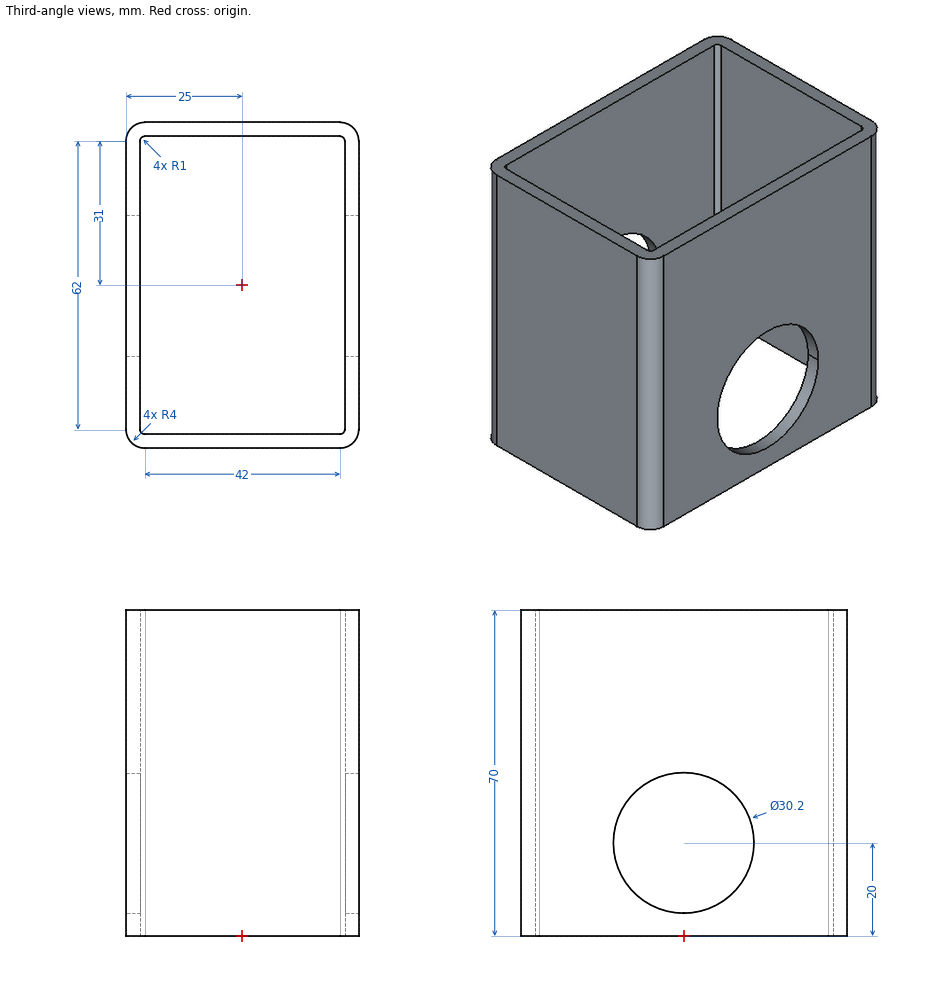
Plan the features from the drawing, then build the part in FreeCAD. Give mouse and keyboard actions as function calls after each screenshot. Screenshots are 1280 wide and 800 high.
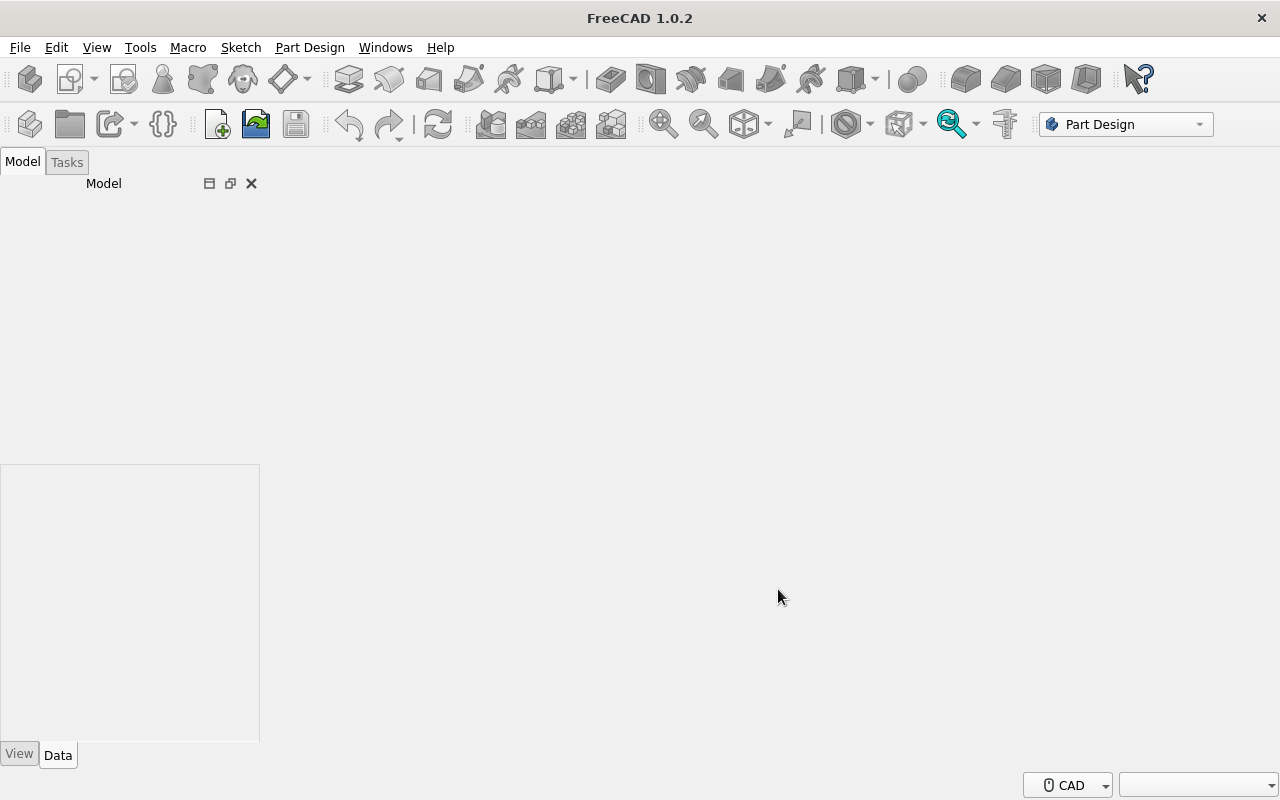
click(216, 124)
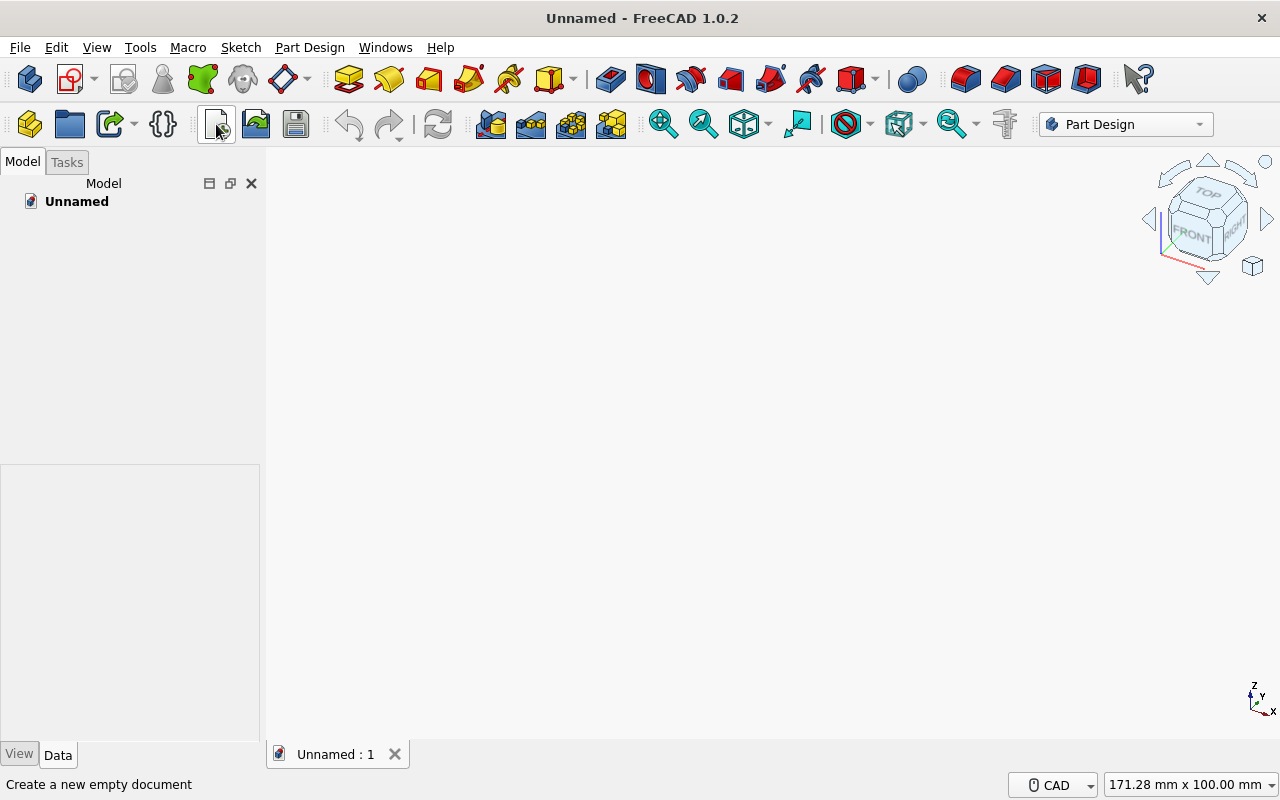
click(70, 80)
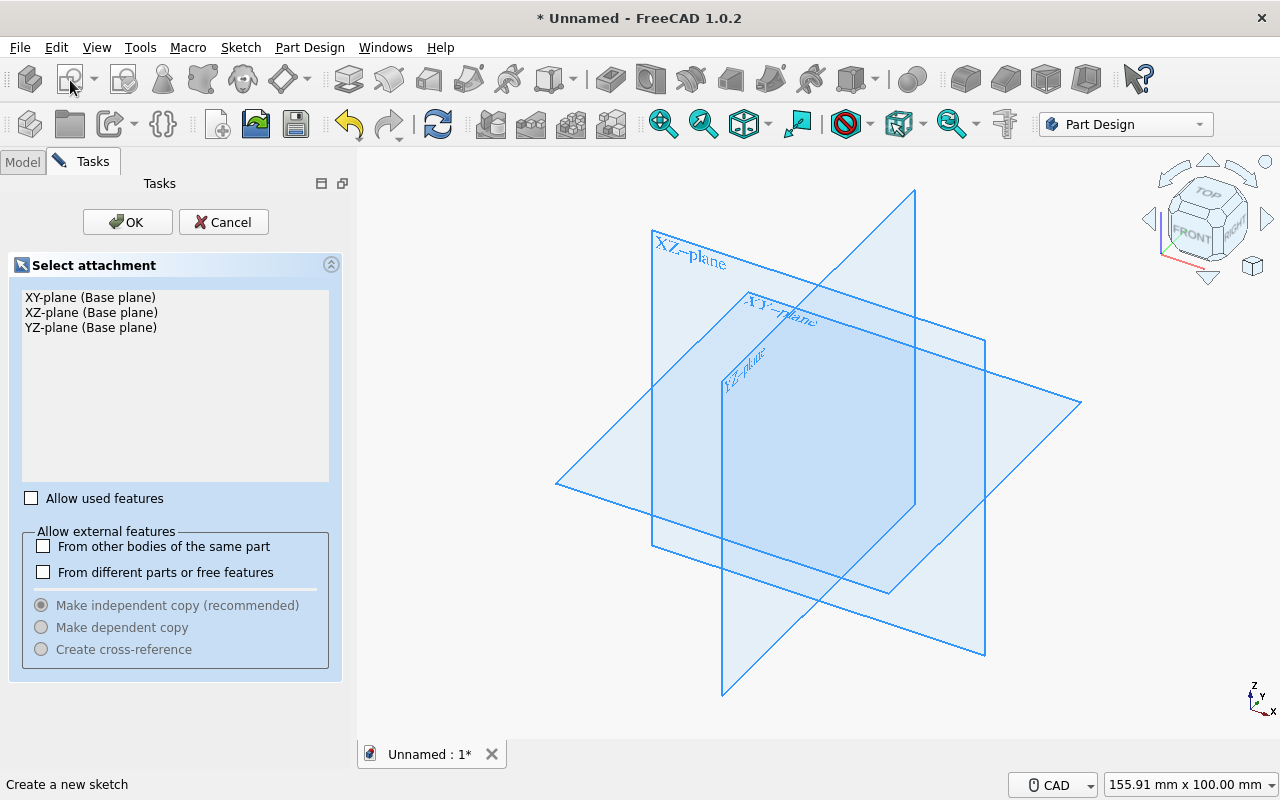
click(82, 298)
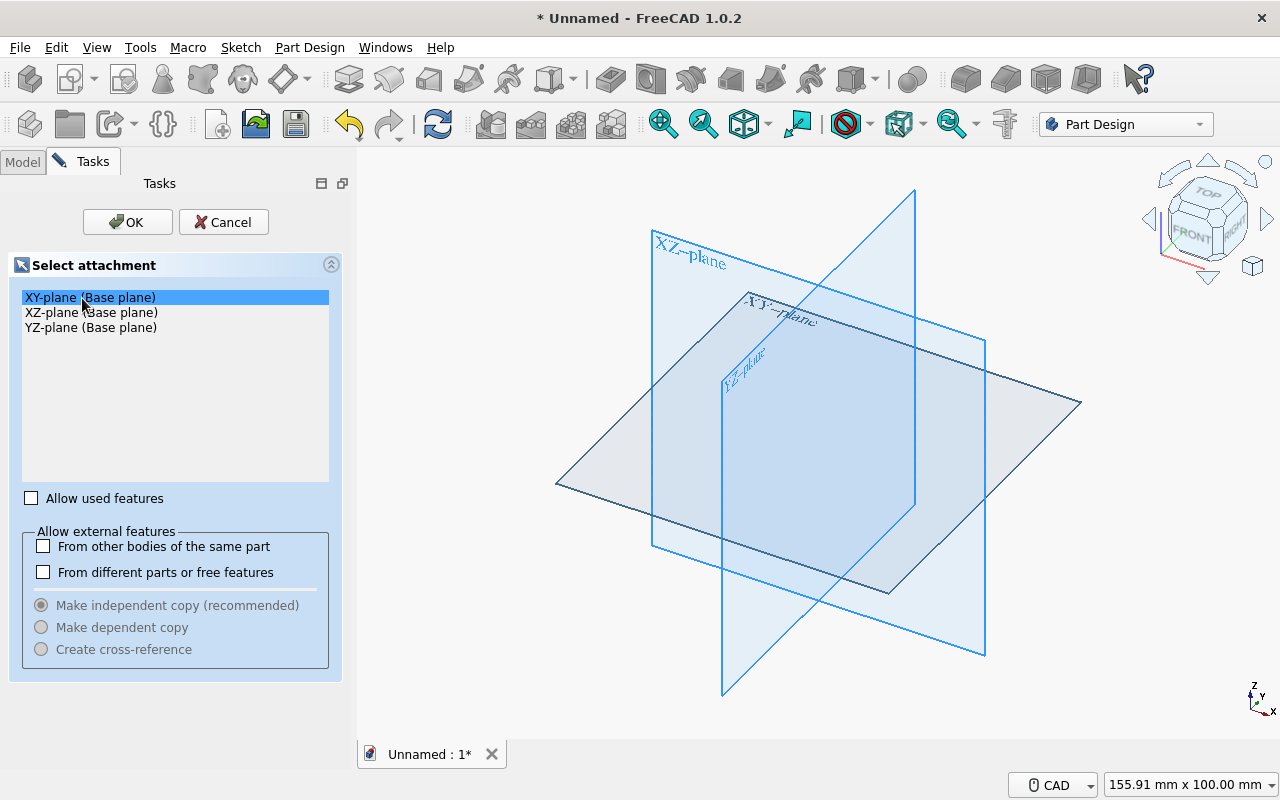
click(128, 222)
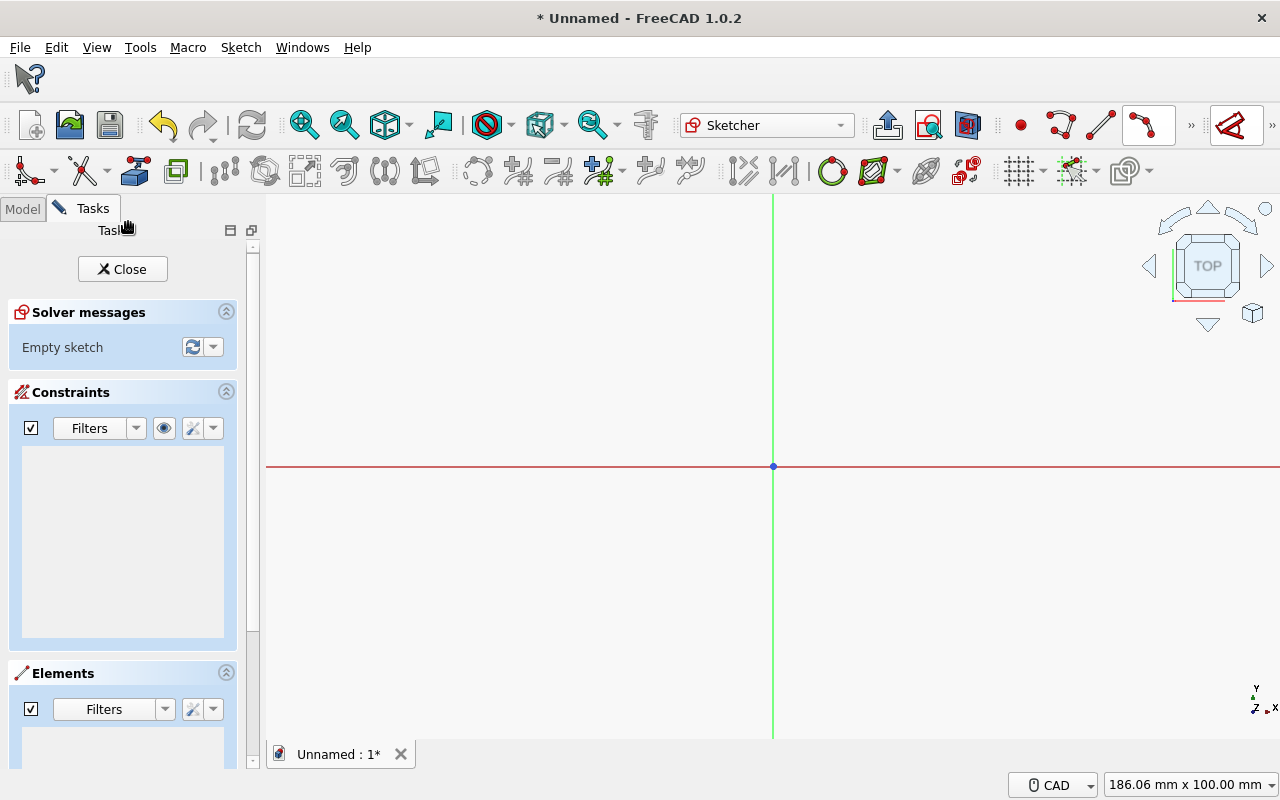
click(1102, 126)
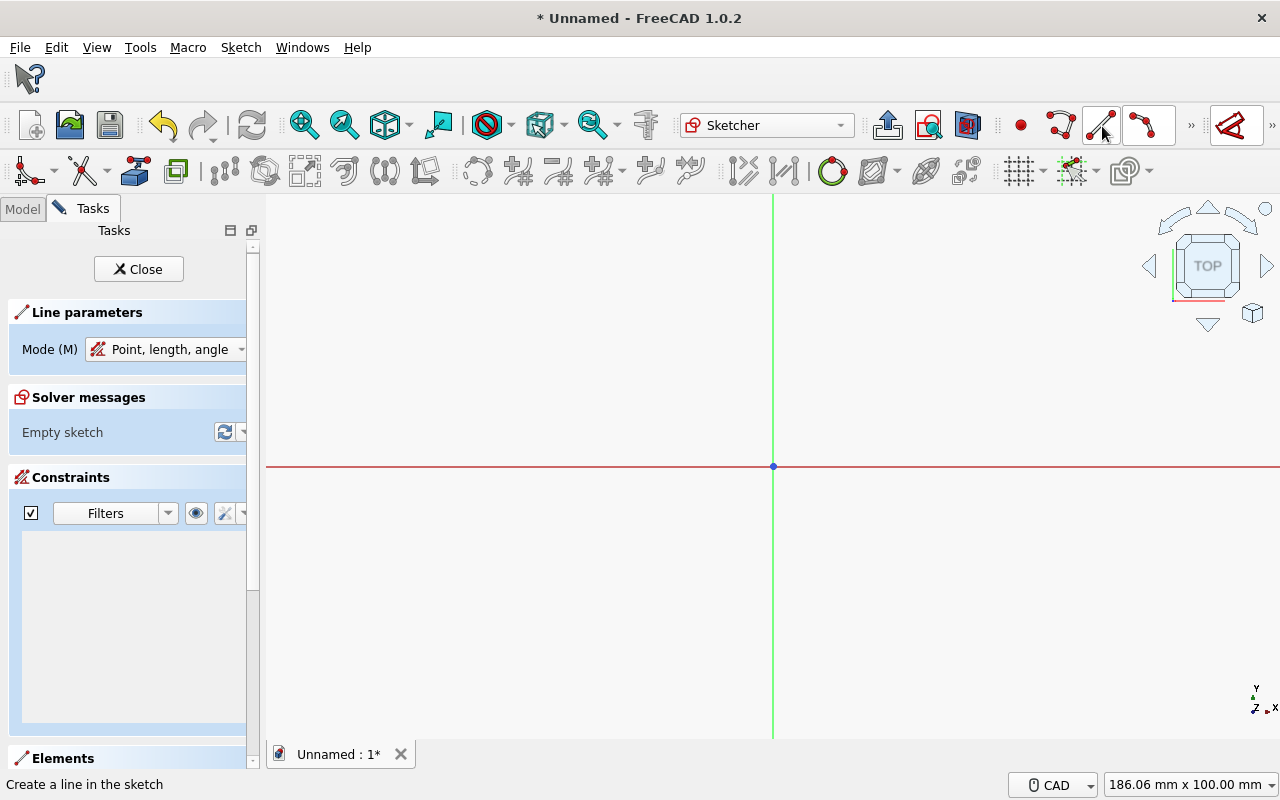
click(637, 298)
click(637, 635)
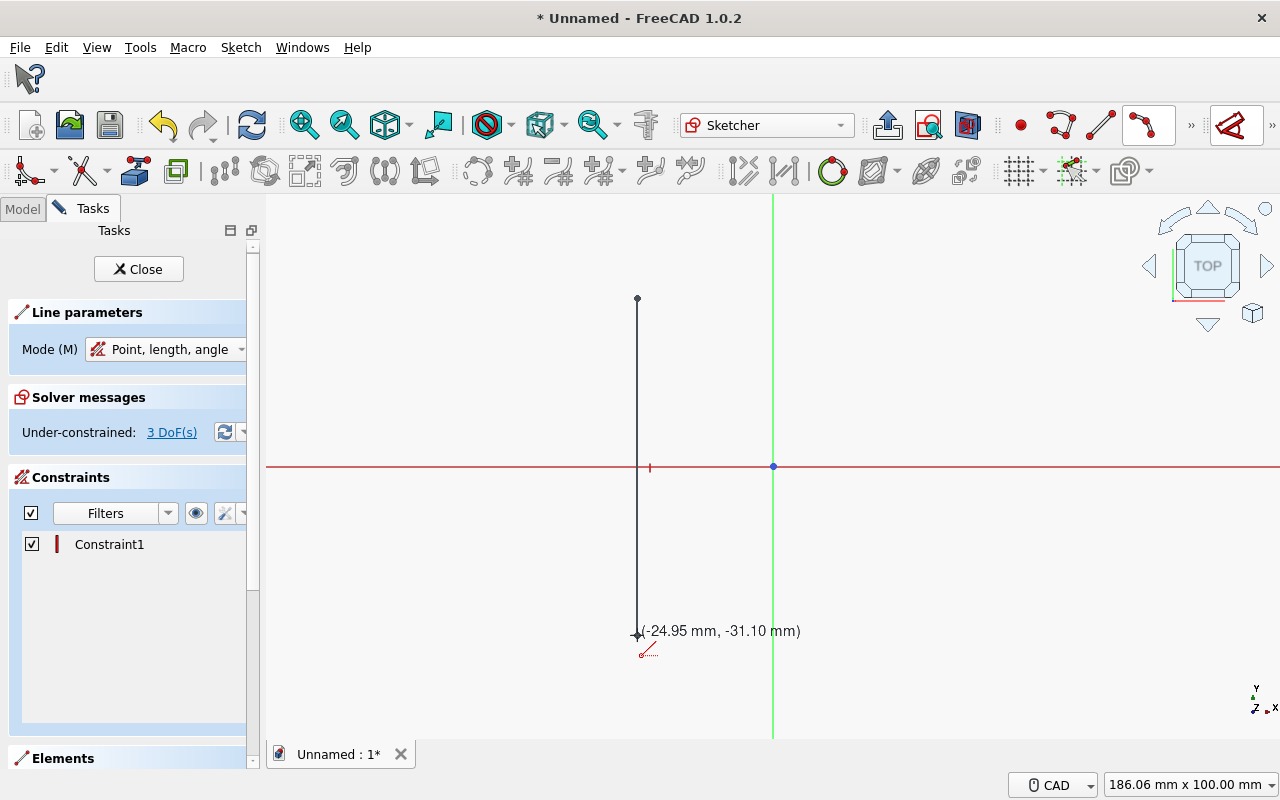
click(659, 657)
click(887, 657)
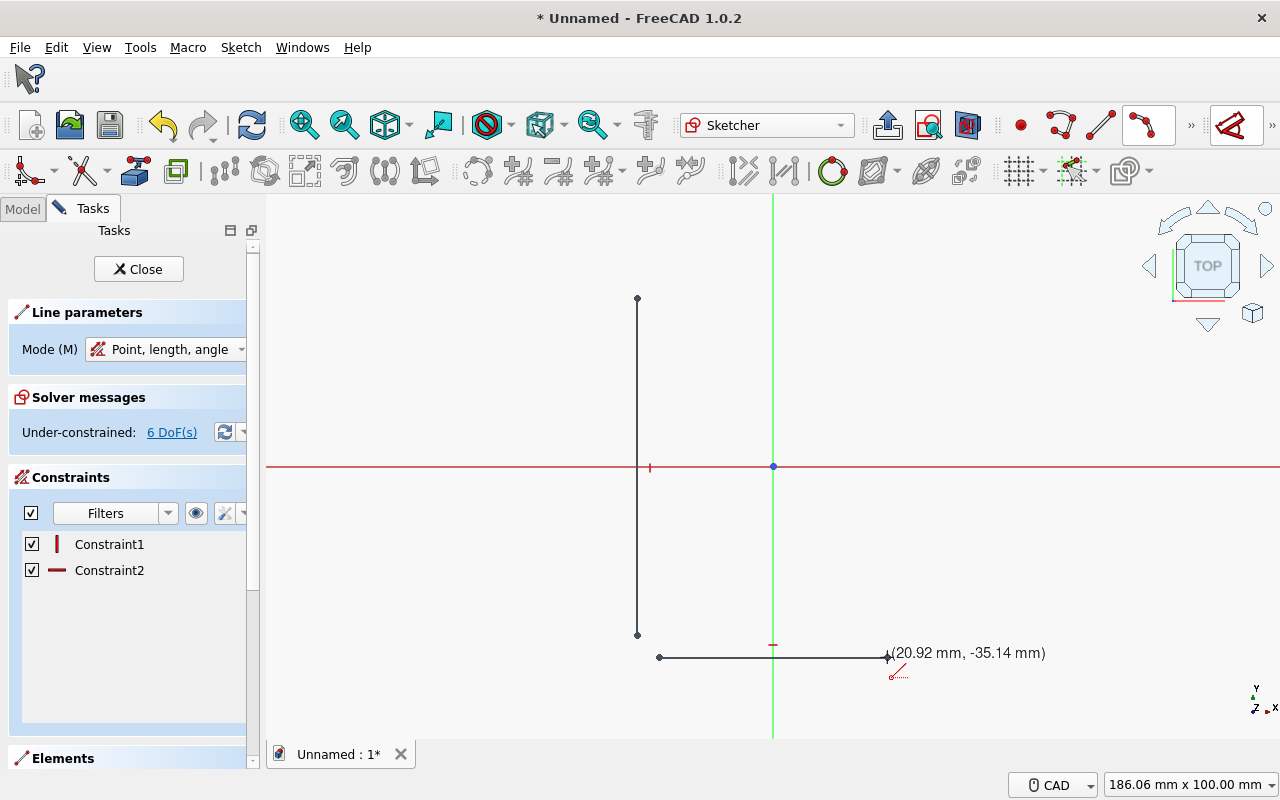
click(909, 635)
click(909, 298)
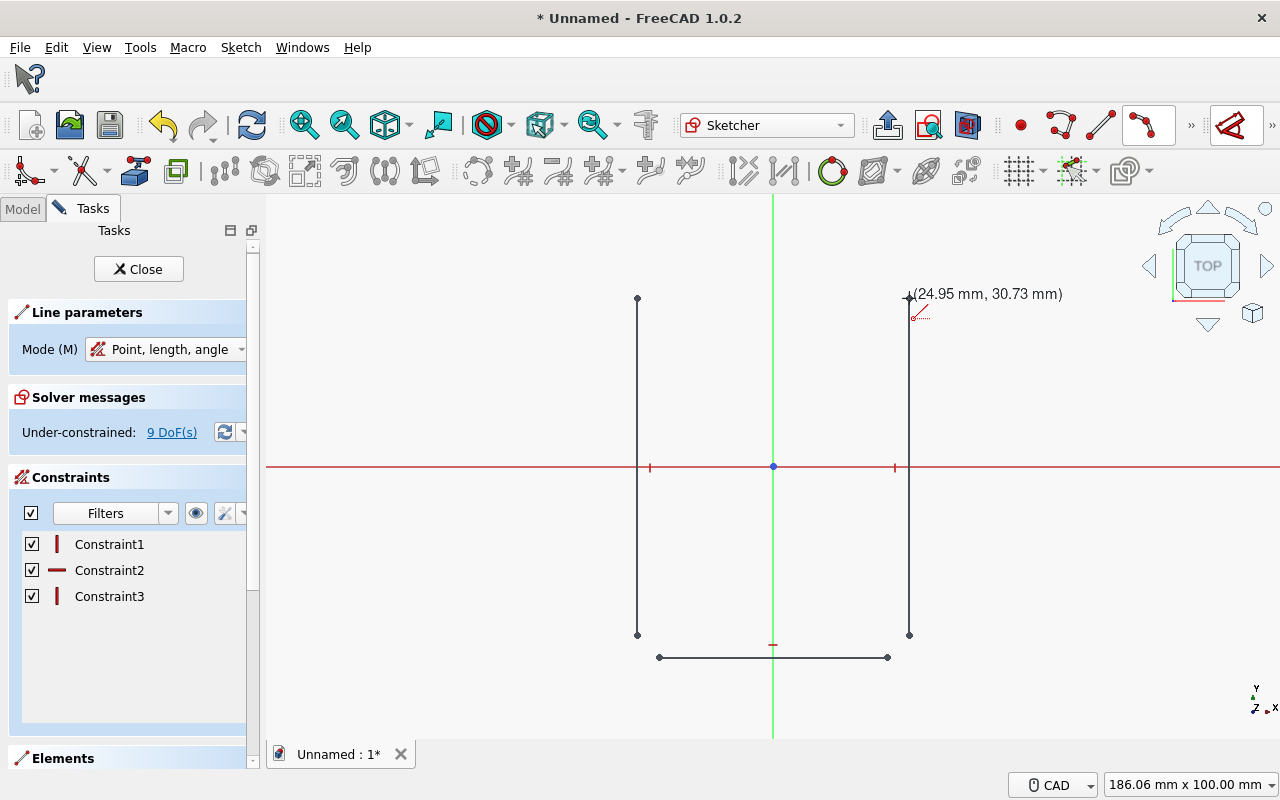
click(887, 276)
click(659, 276)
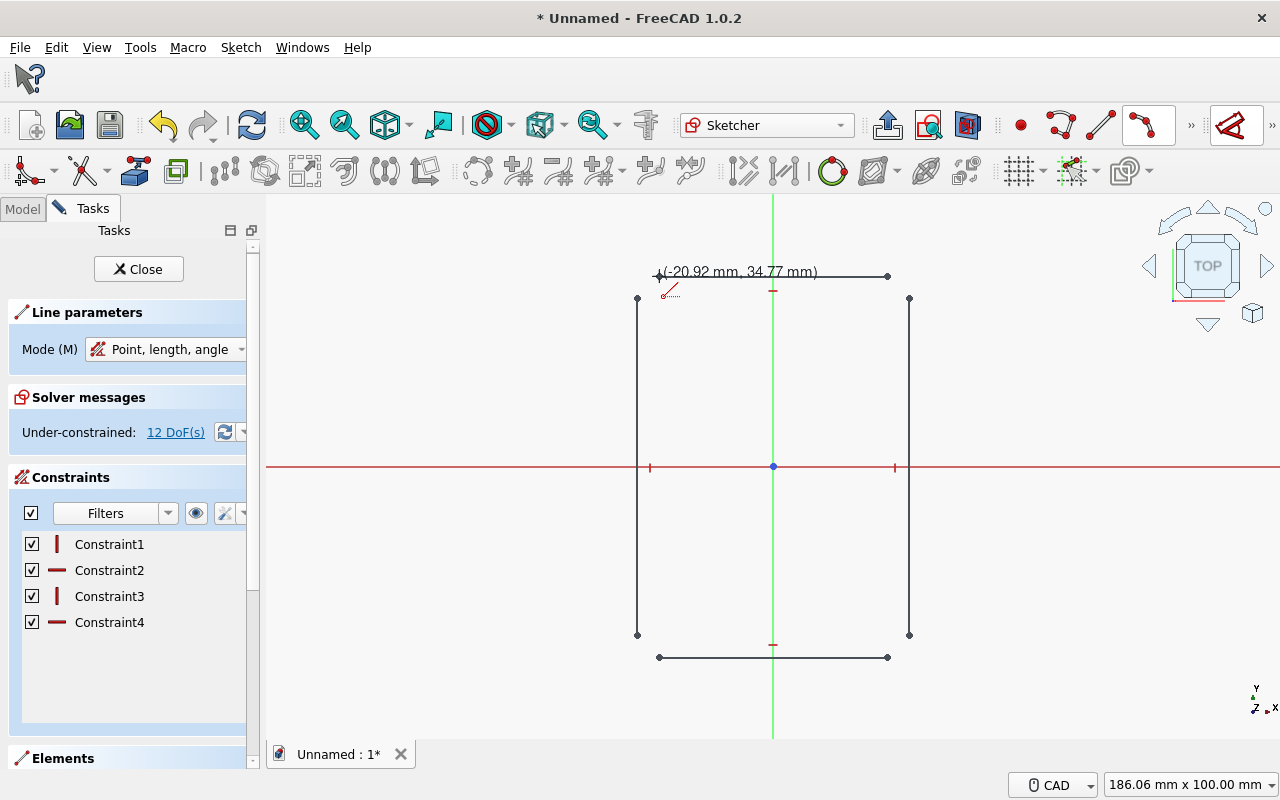
click(1142, 126)